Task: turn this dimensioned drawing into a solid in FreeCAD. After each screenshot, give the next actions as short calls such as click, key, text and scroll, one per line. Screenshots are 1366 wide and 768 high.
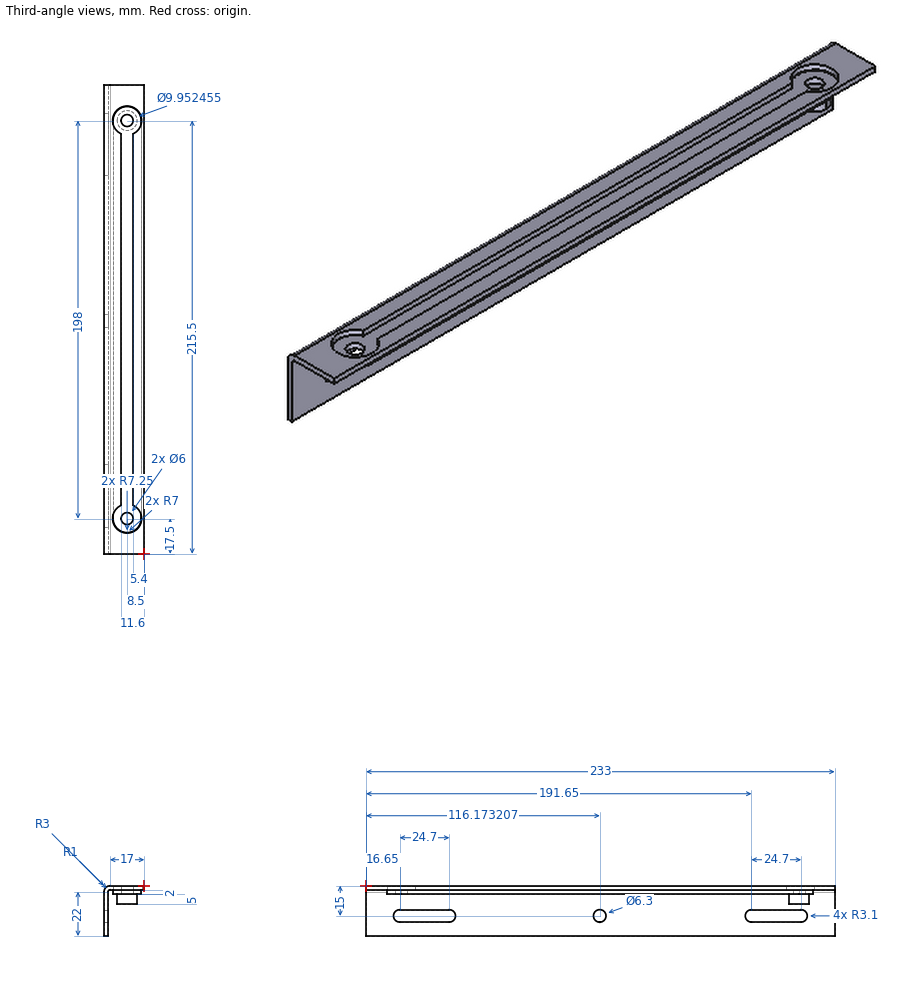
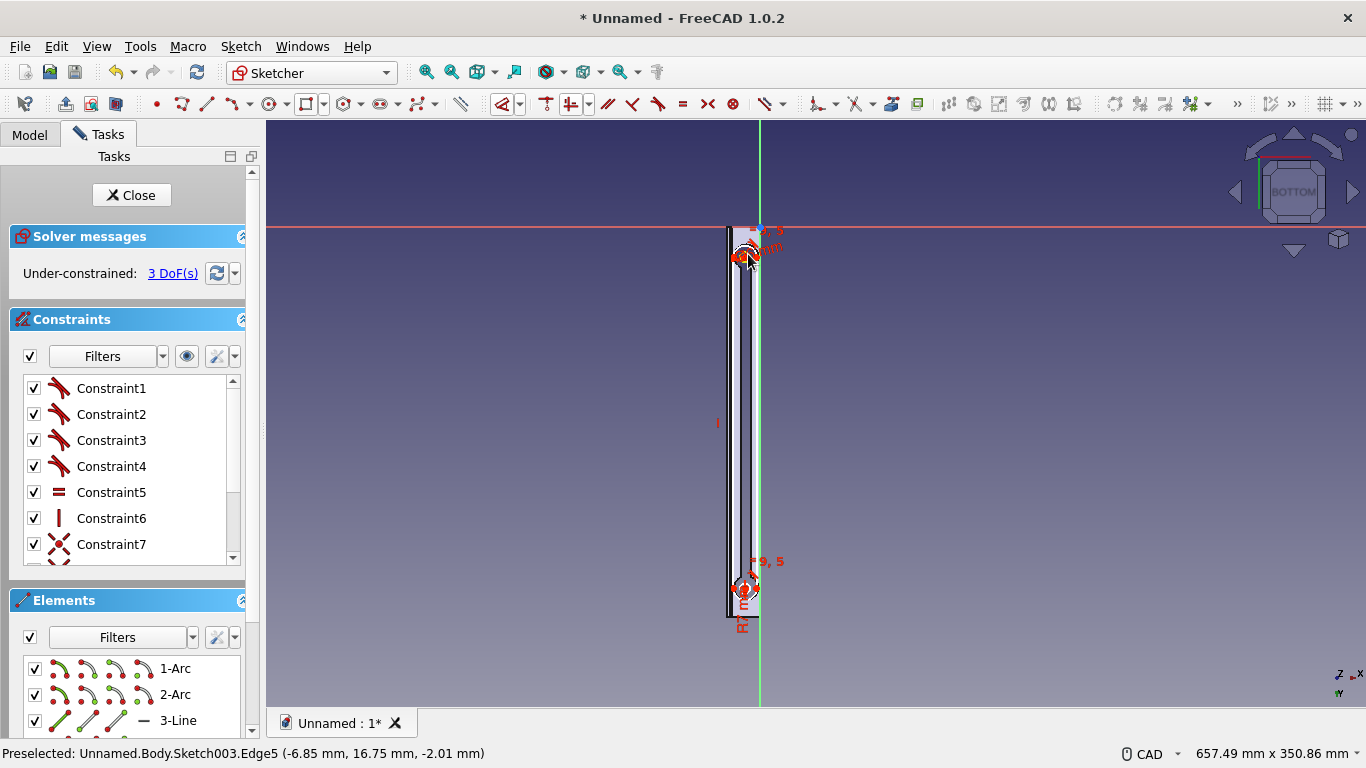
click(733, 357)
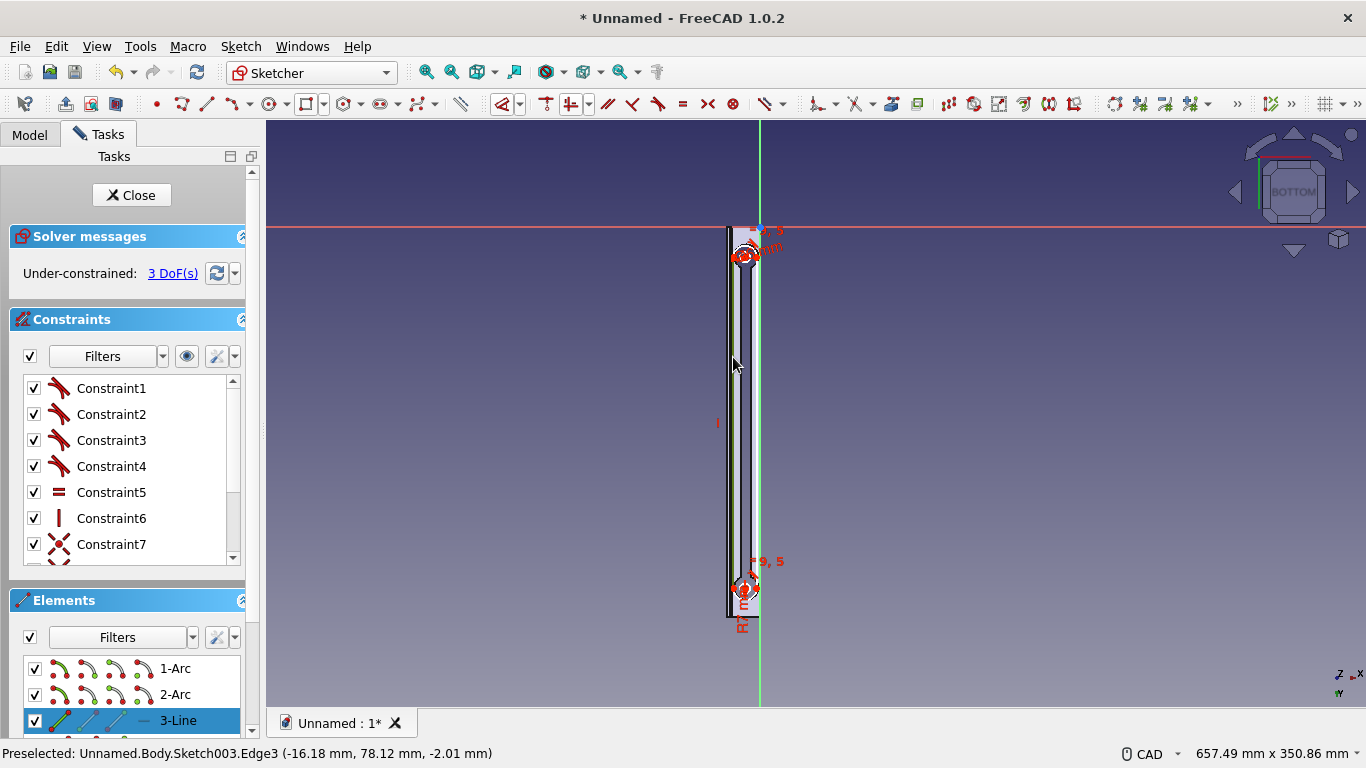
key(i)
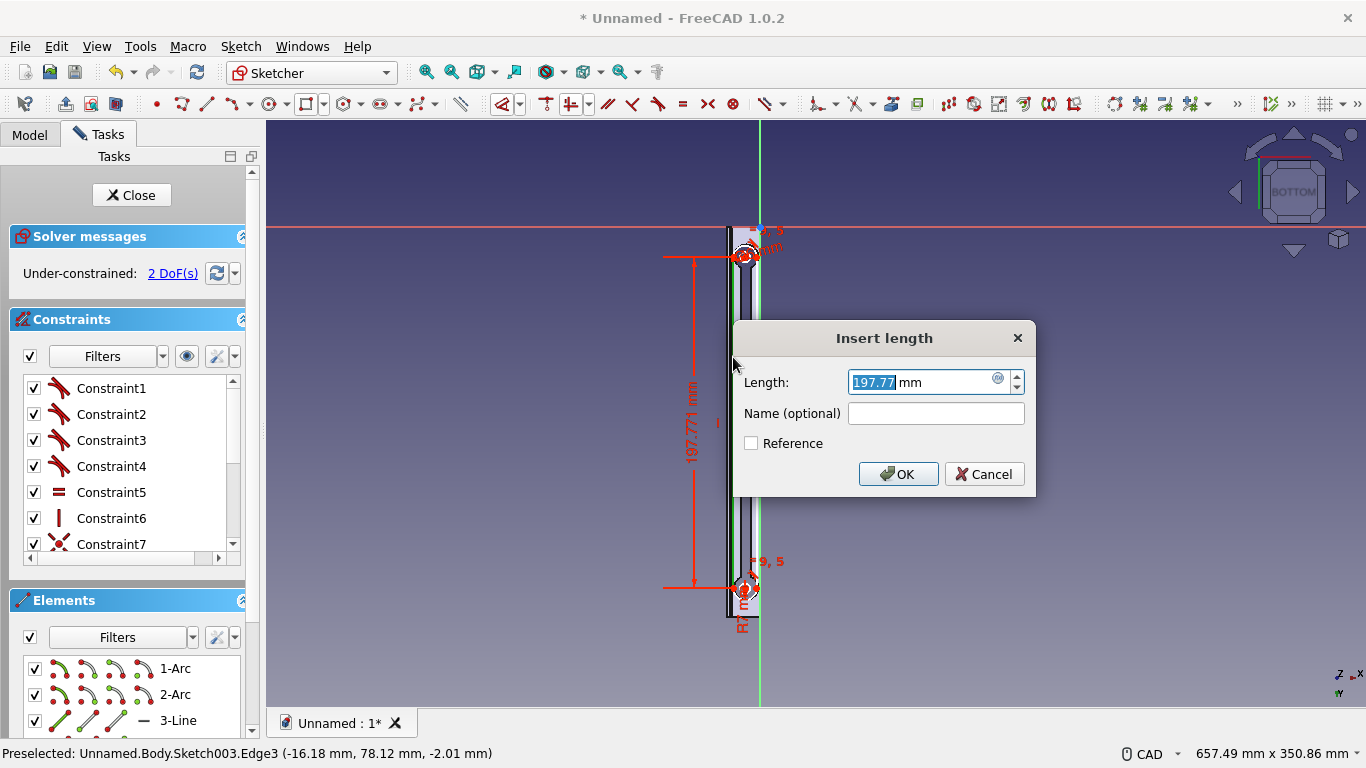
text(198)
key(Return)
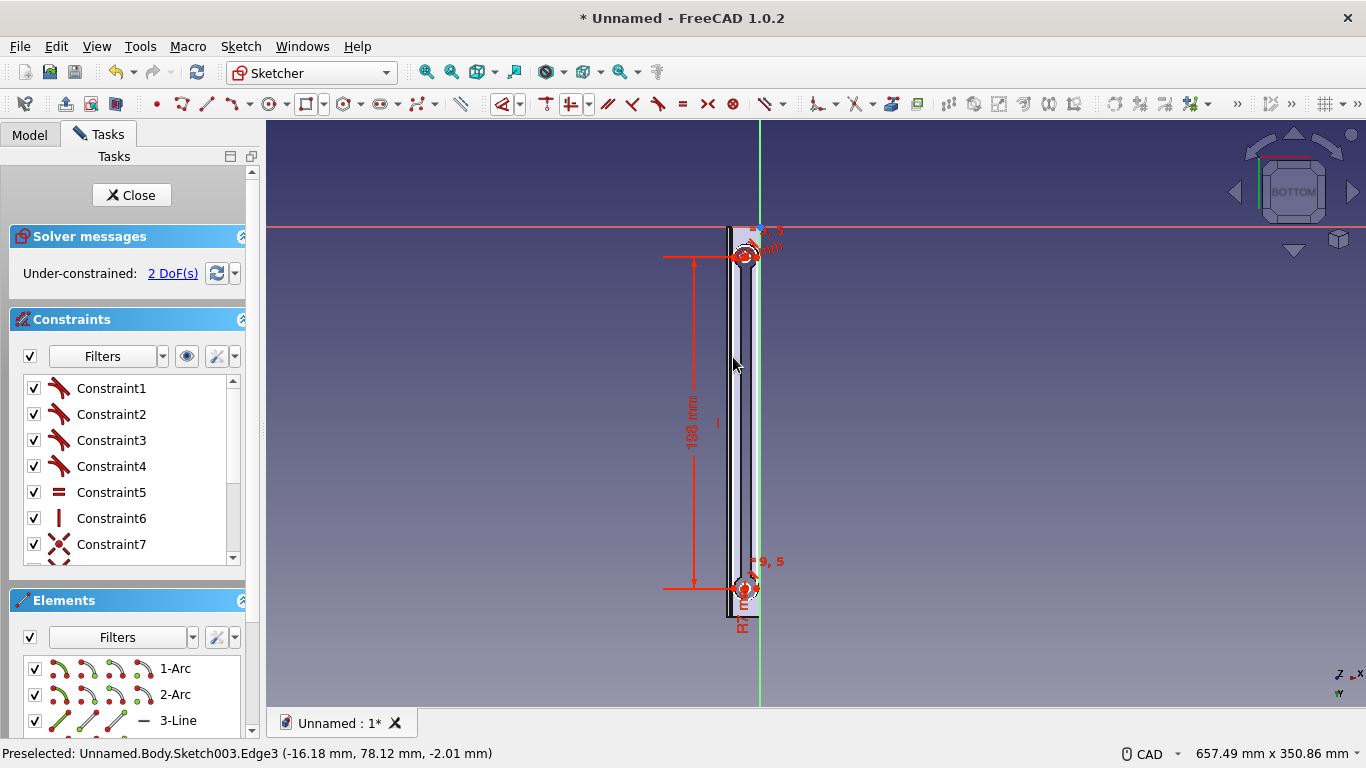
scroll(745, 257, up, 6)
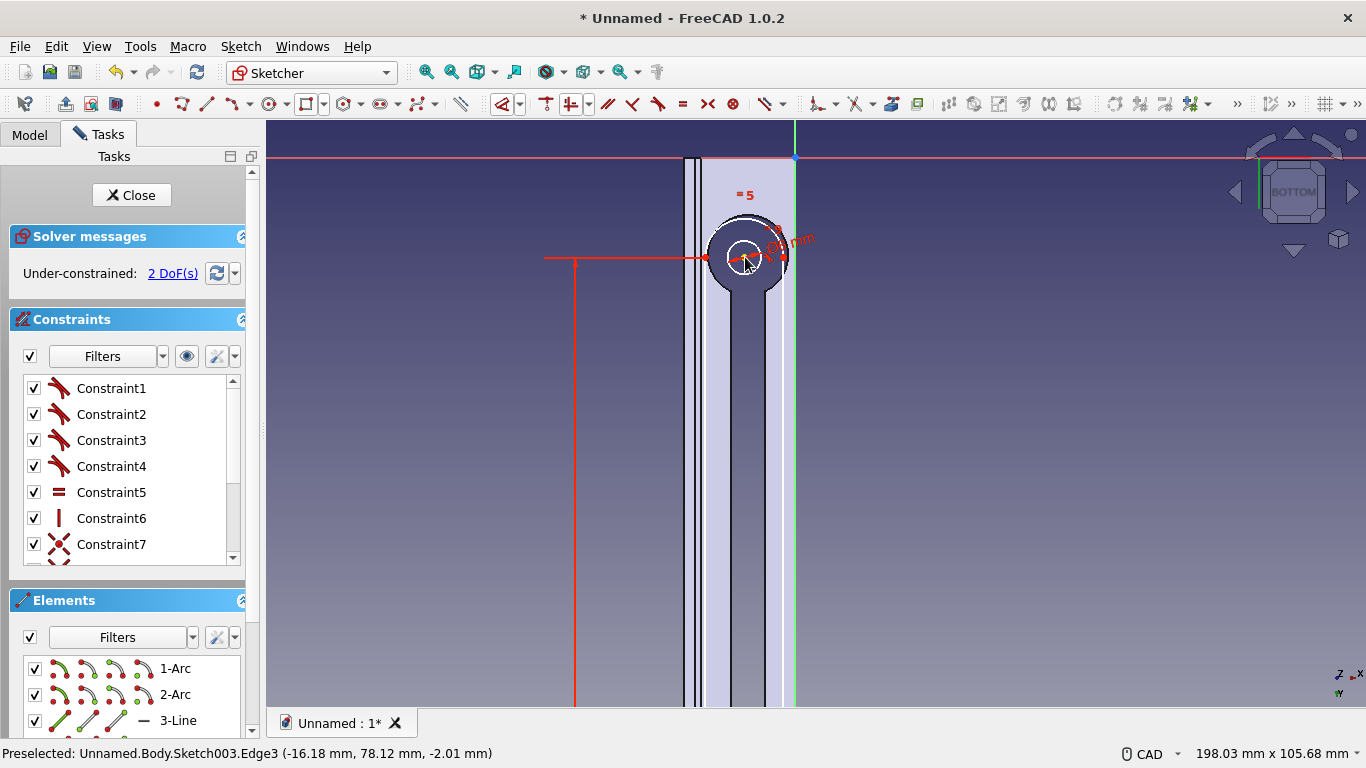
click(744, 258)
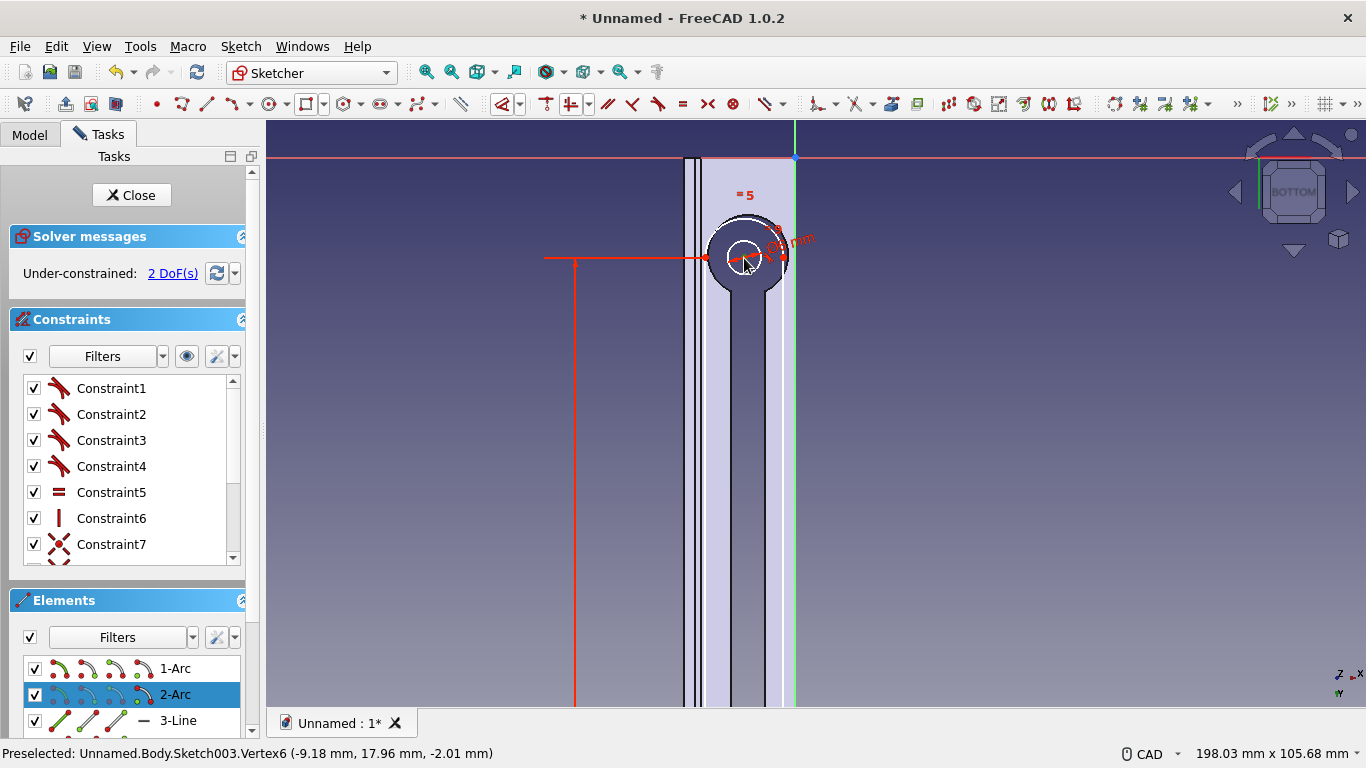
key(l)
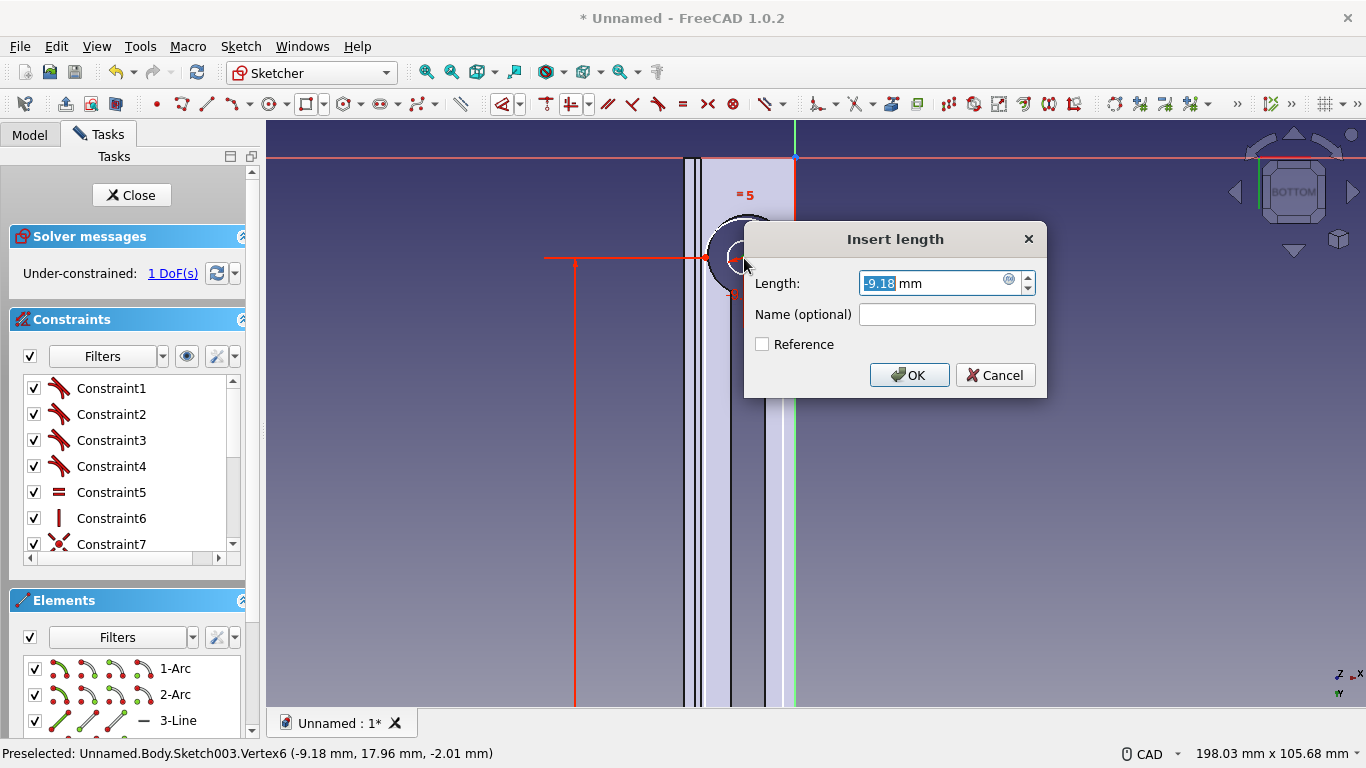
text(-8.5)
key(Return)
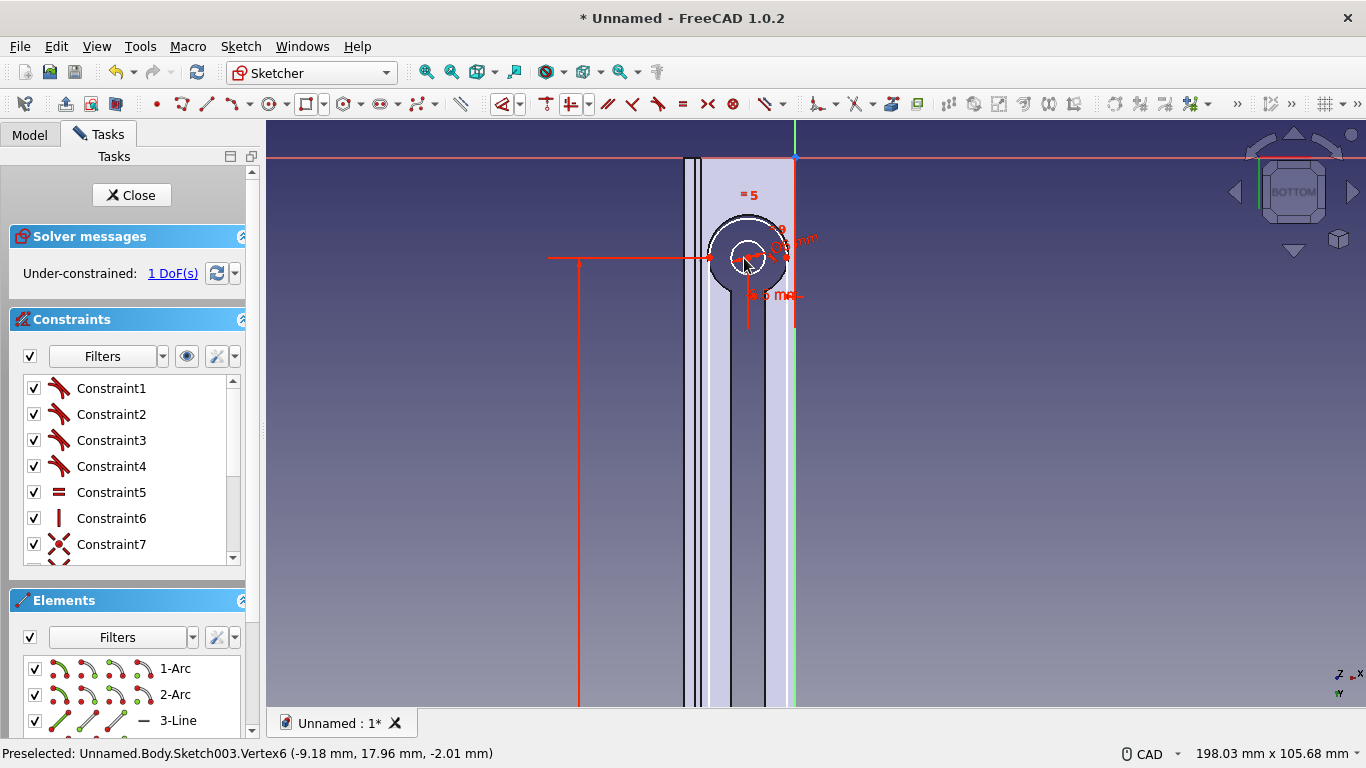
click(748, 258)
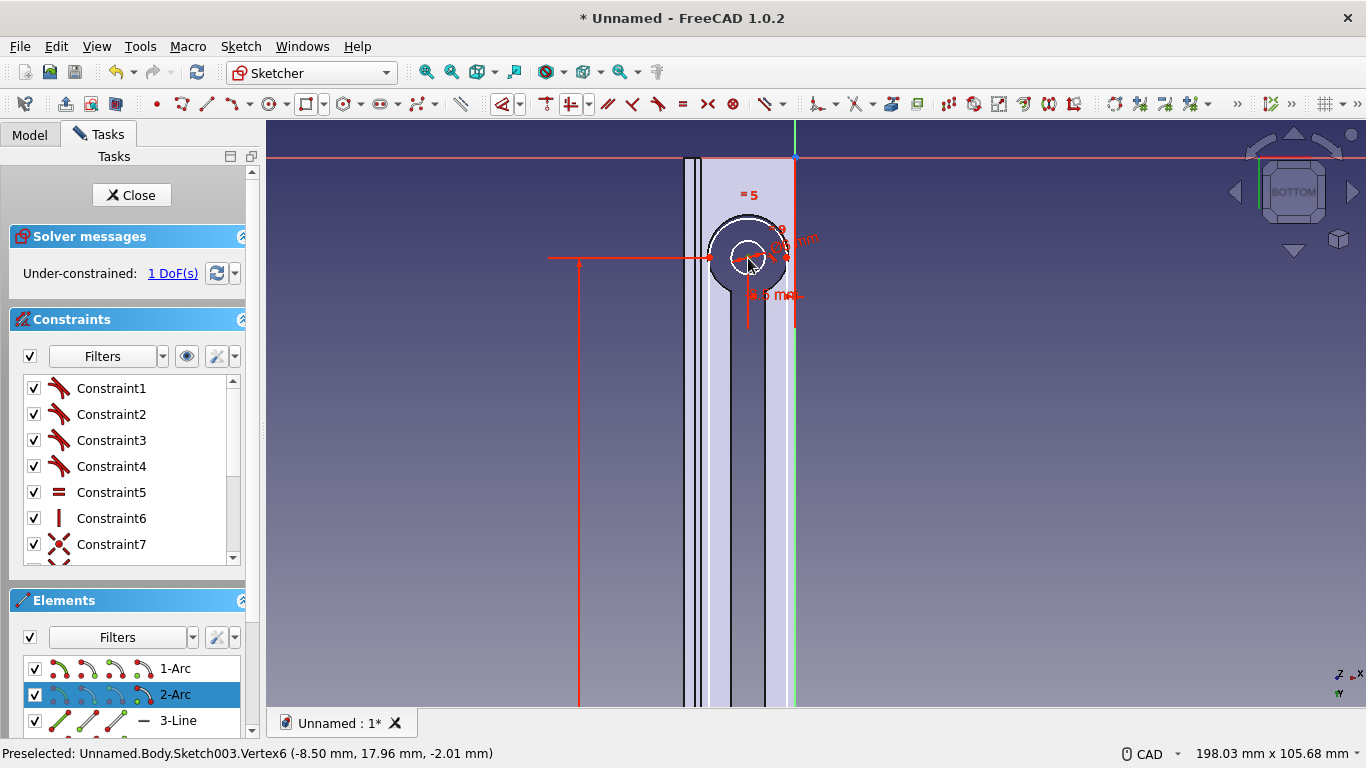
key(i)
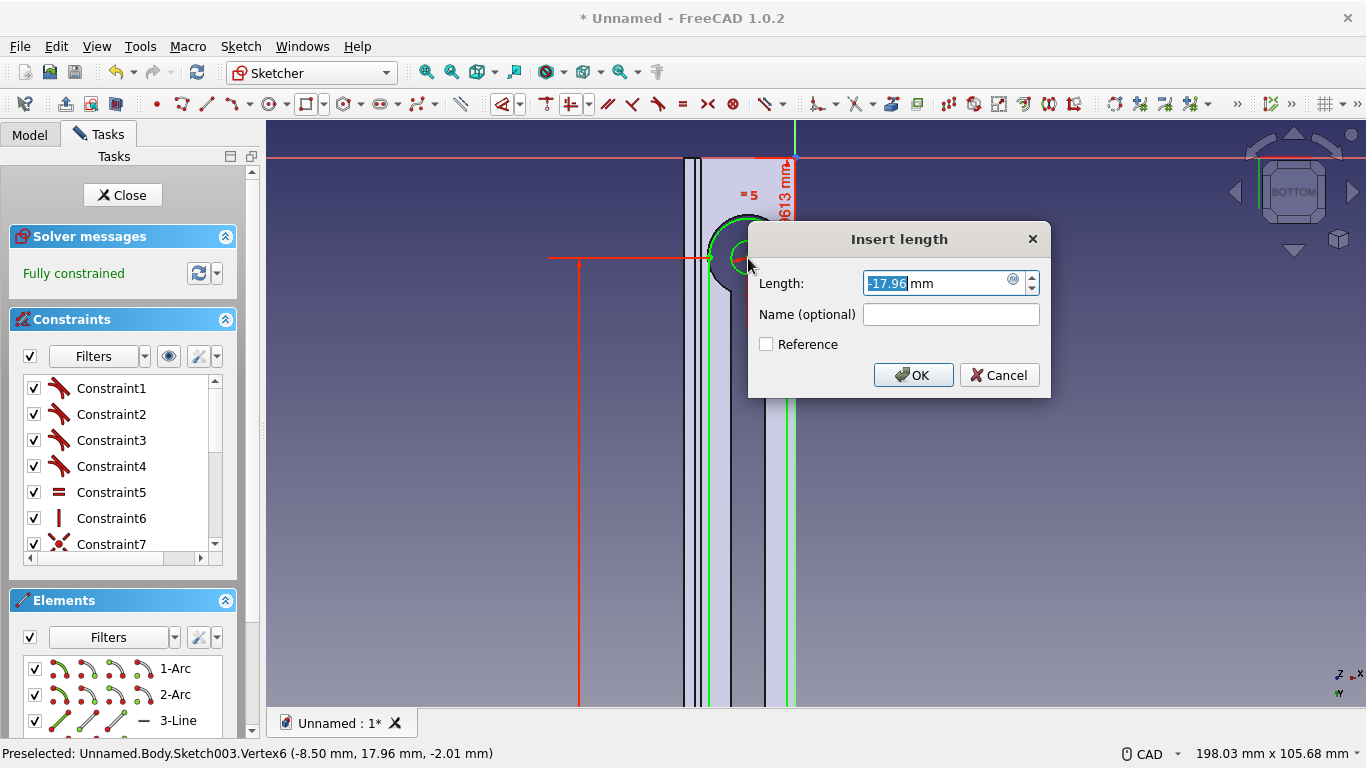
text(-17.5)
key(Return)